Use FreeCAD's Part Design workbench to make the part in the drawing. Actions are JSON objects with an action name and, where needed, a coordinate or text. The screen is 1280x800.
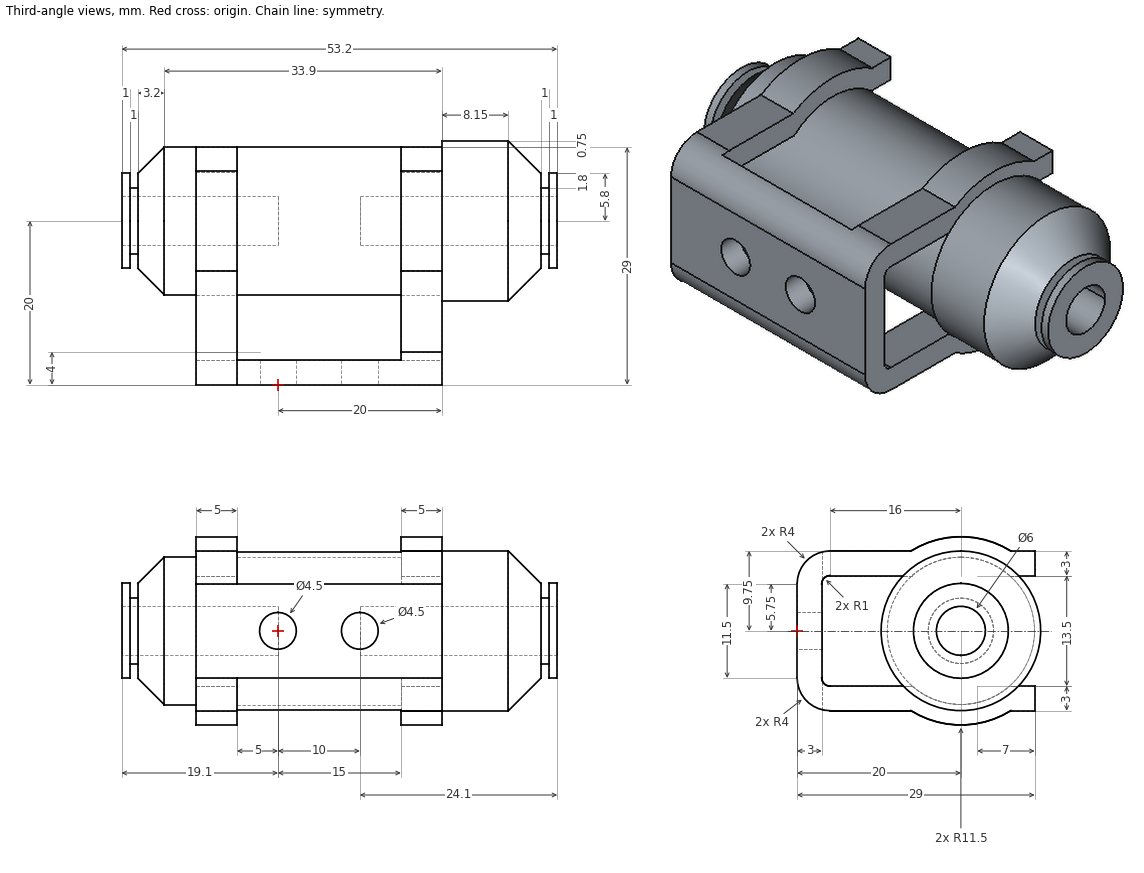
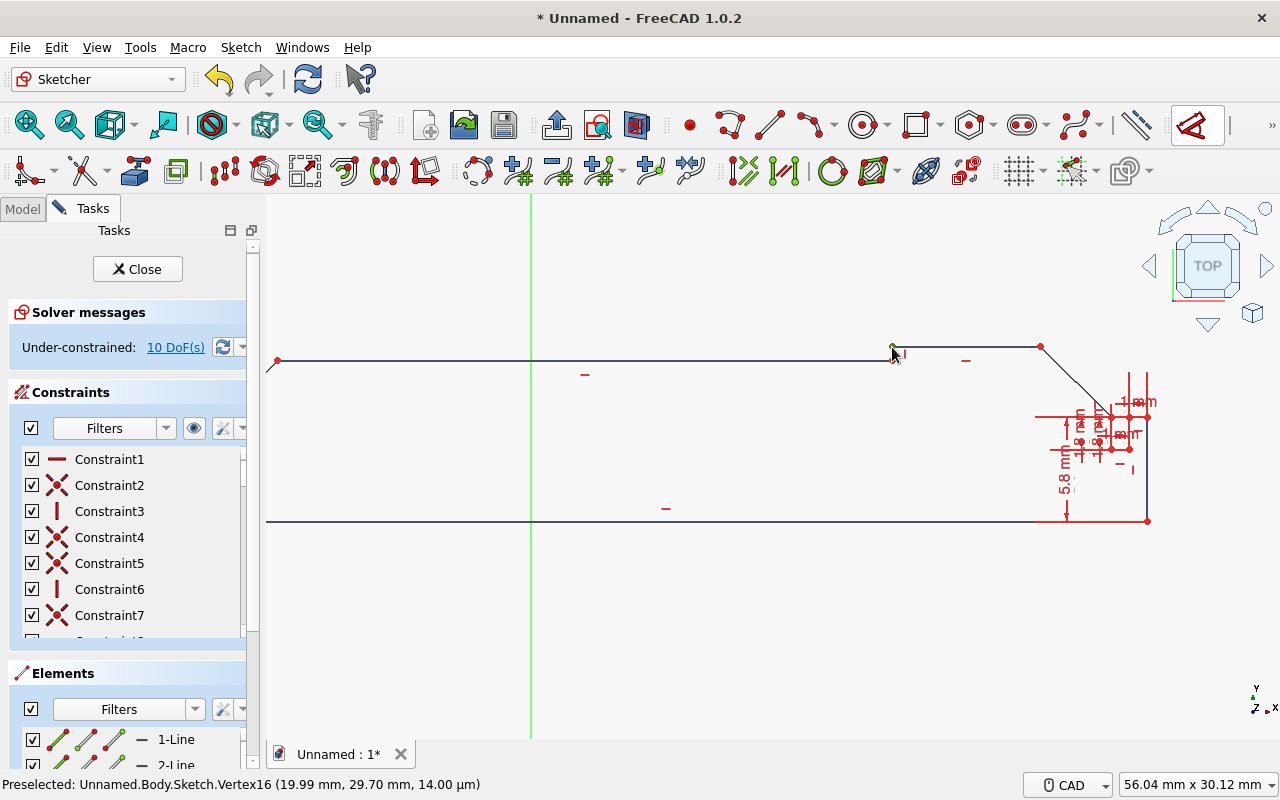
{"action": "left_click", "coordinate": [1218, 126]}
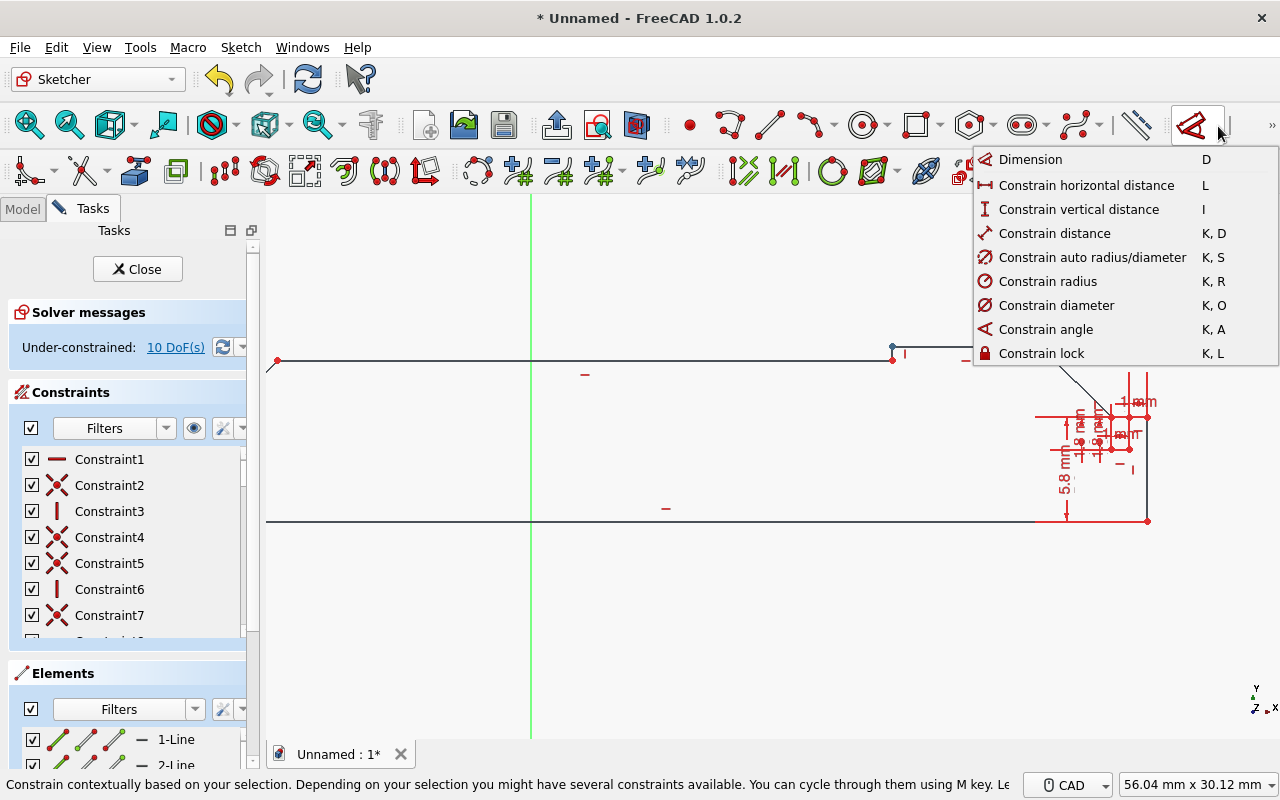
{"action": "left_click", "coordinate": [1126, 185]}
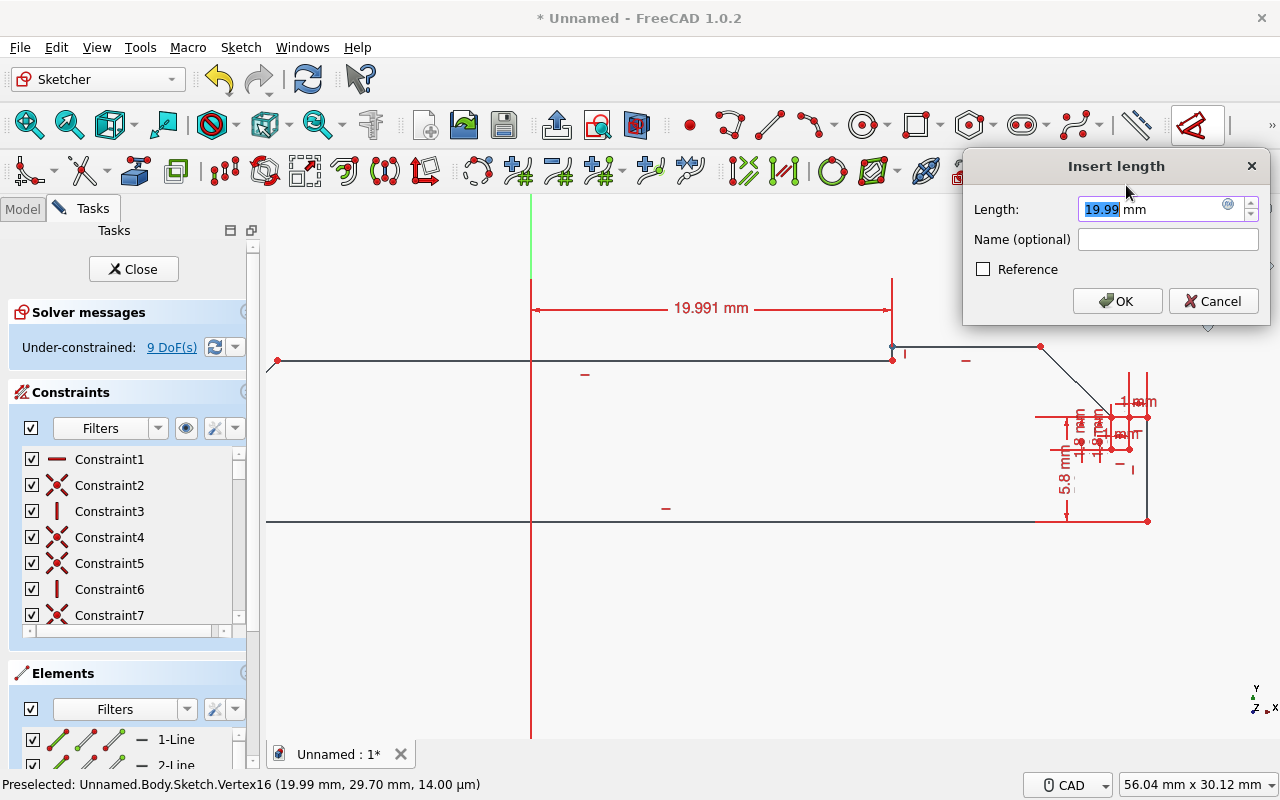
{"action": "type", "text": "20"}
{"action": "key", "text": "Return"}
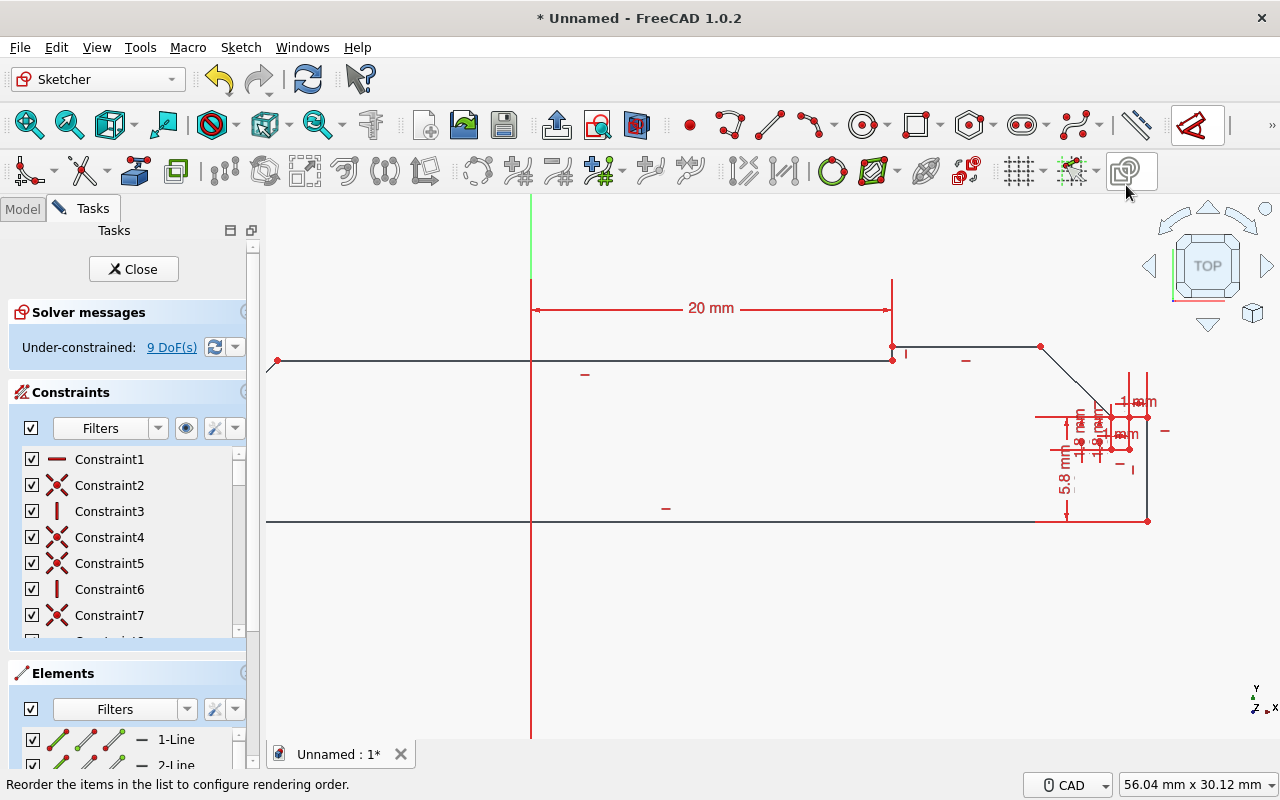
{"action": "left_click", "coordinate": [892, 361]}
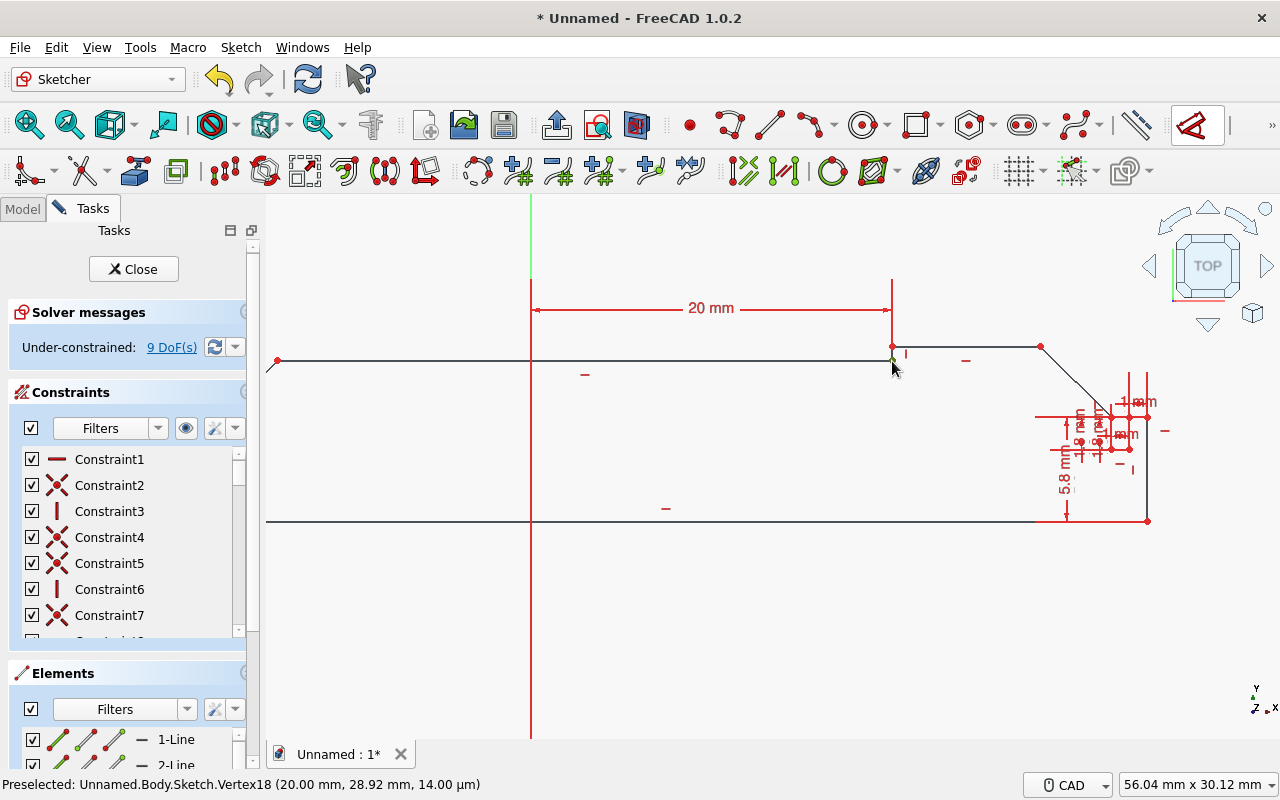
{"action": "left_click", "coordinate": [1218, 126]}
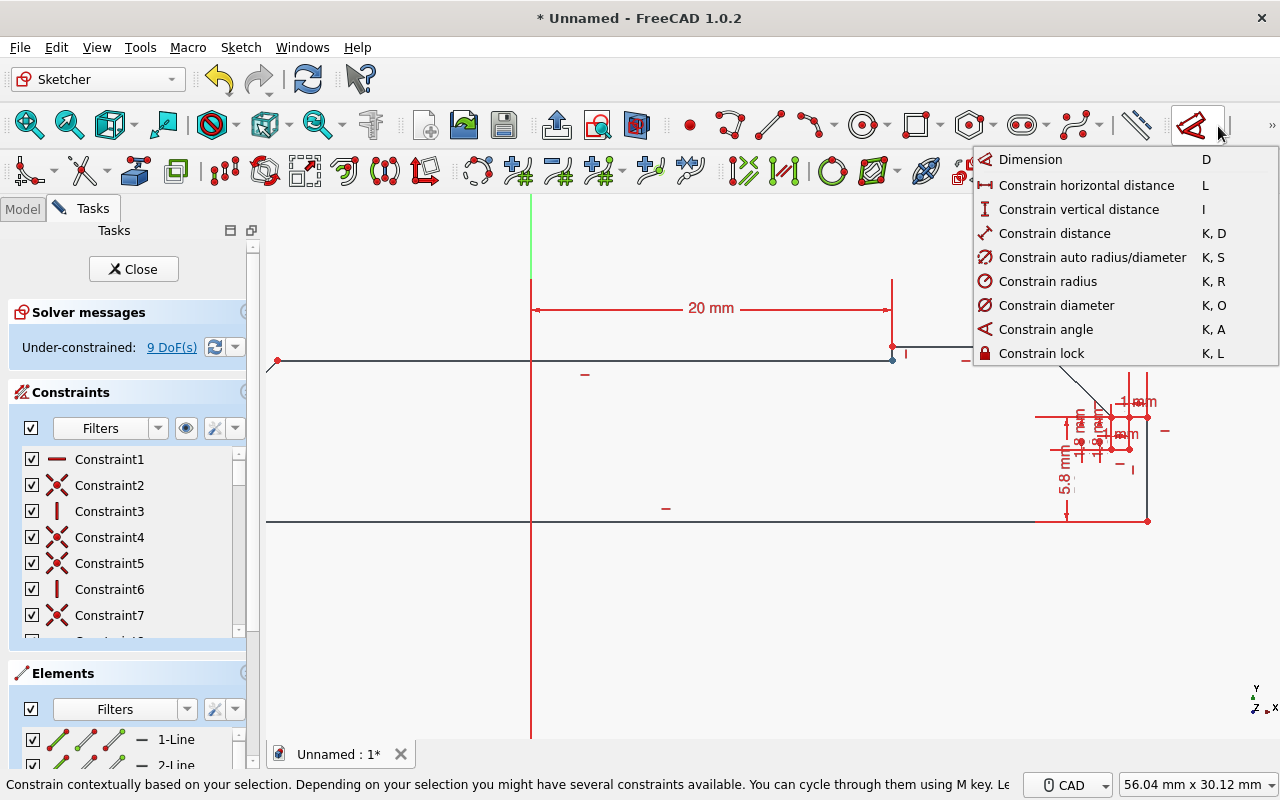
{"action": "left_click", "coordinate": [1126, 209]}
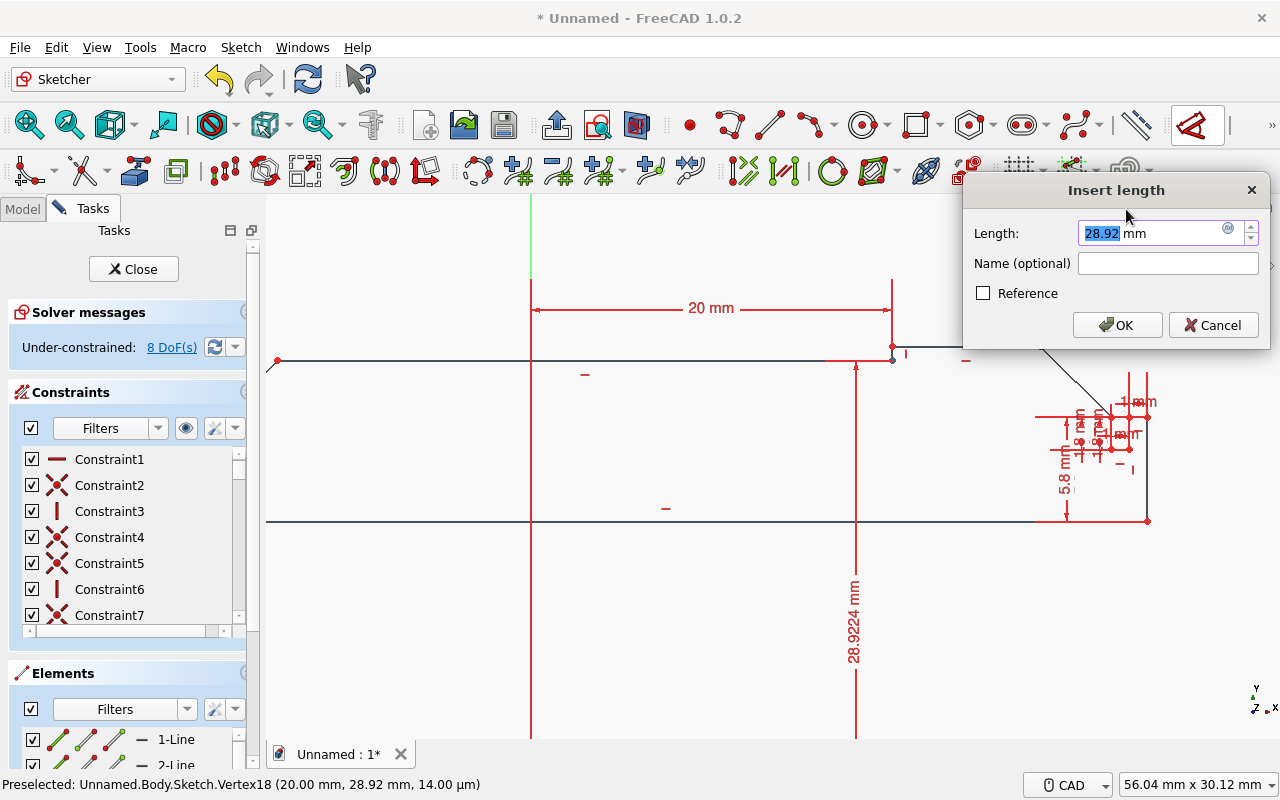
{"action": "type", "text": "29"}
{"action": "key", "text": "Return"}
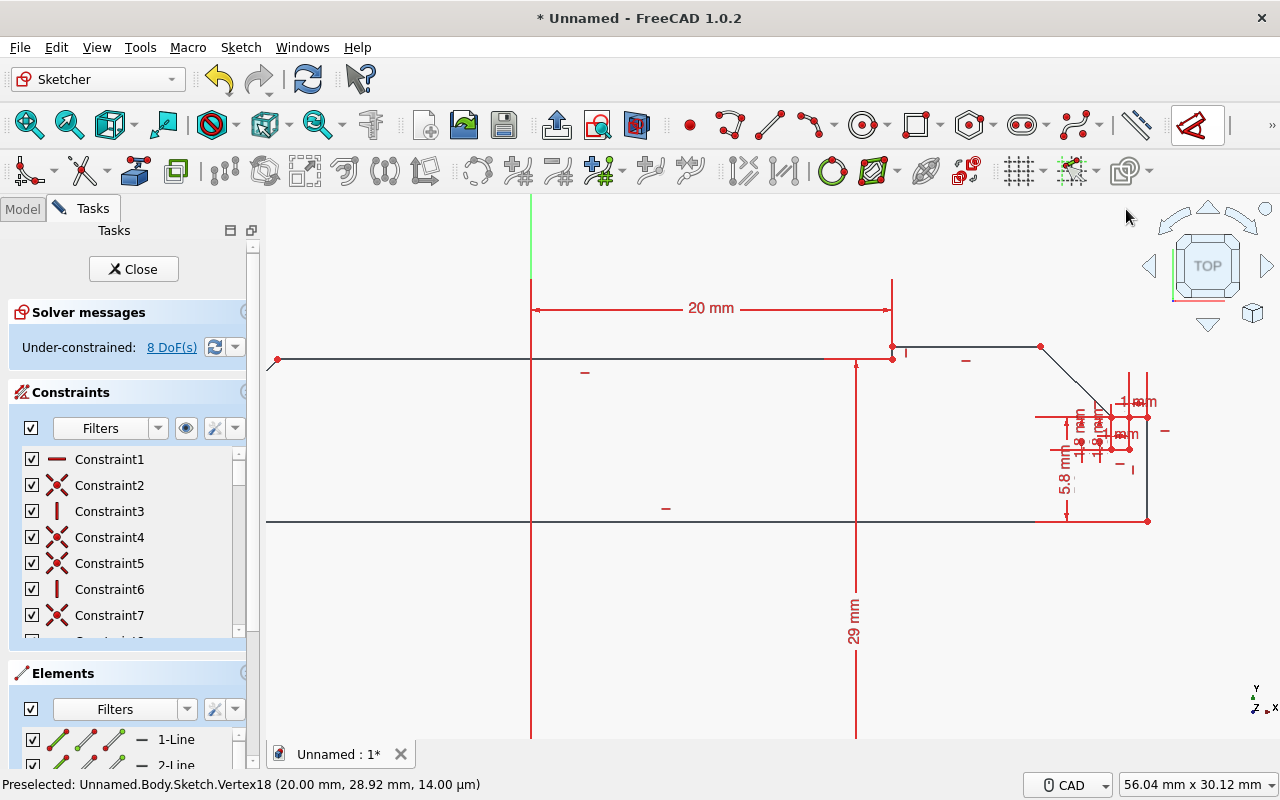
{"action": "scroll", "coordinate": [893, 346], "scroll_direction": "down", "scroll_amount": 4}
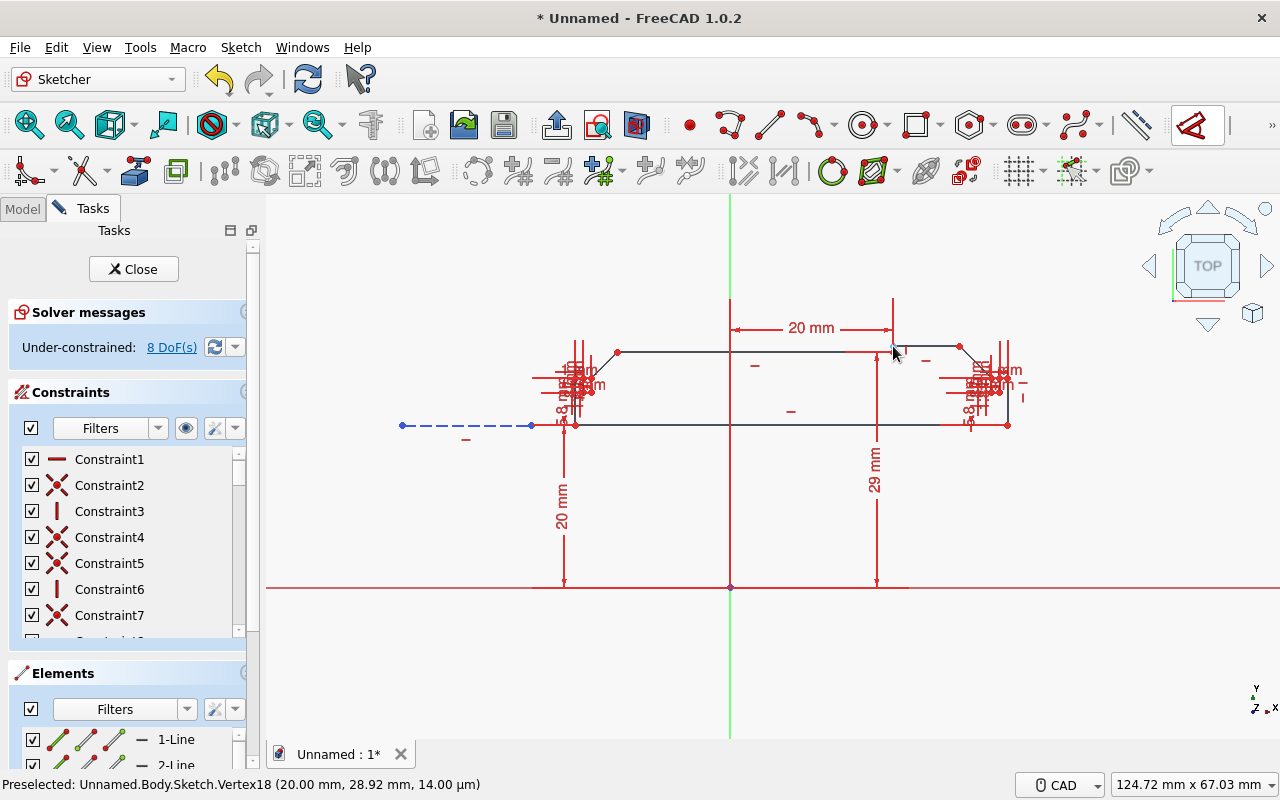
{"action": "left_click", "coordinate": [532, 426]}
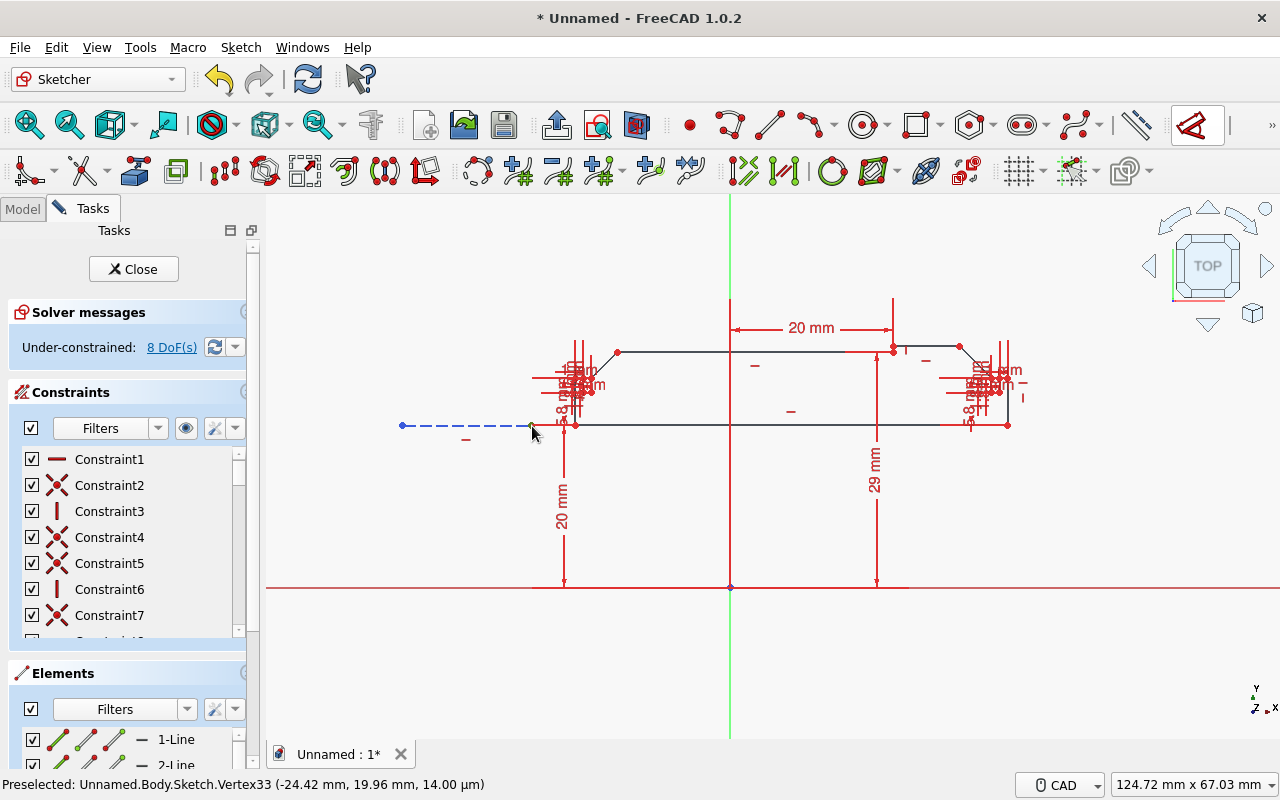
{"action": "key", "text": "i"}